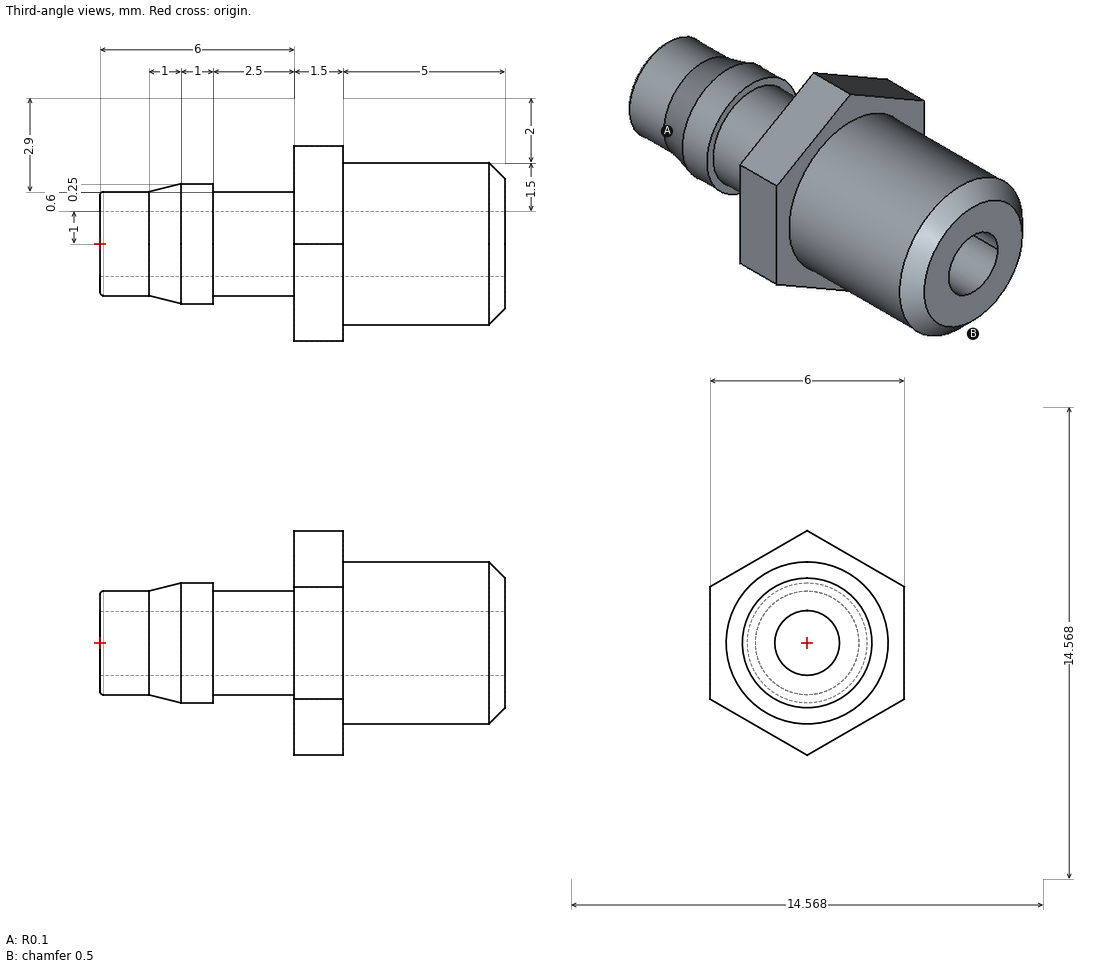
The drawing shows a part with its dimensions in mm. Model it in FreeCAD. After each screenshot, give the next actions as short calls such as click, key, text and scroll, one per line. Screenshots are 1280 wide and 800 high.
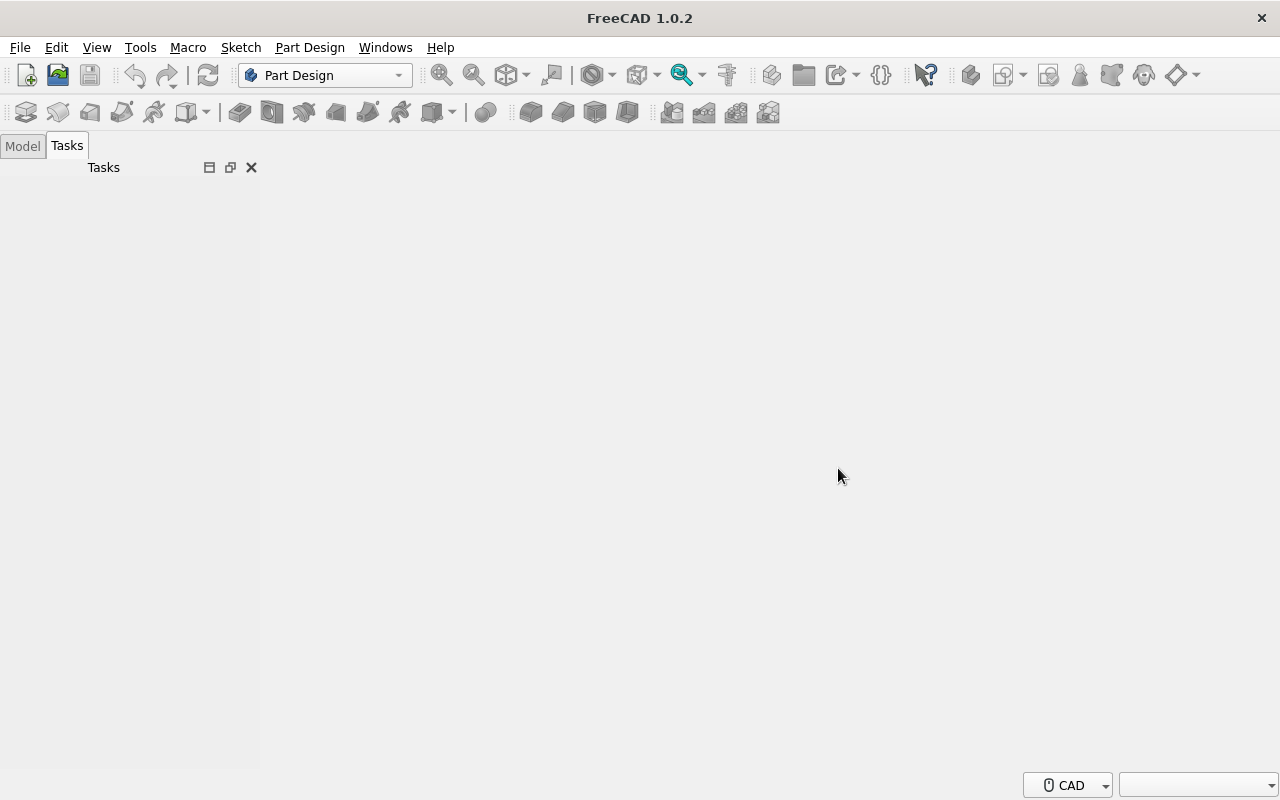
key(ctrl+n)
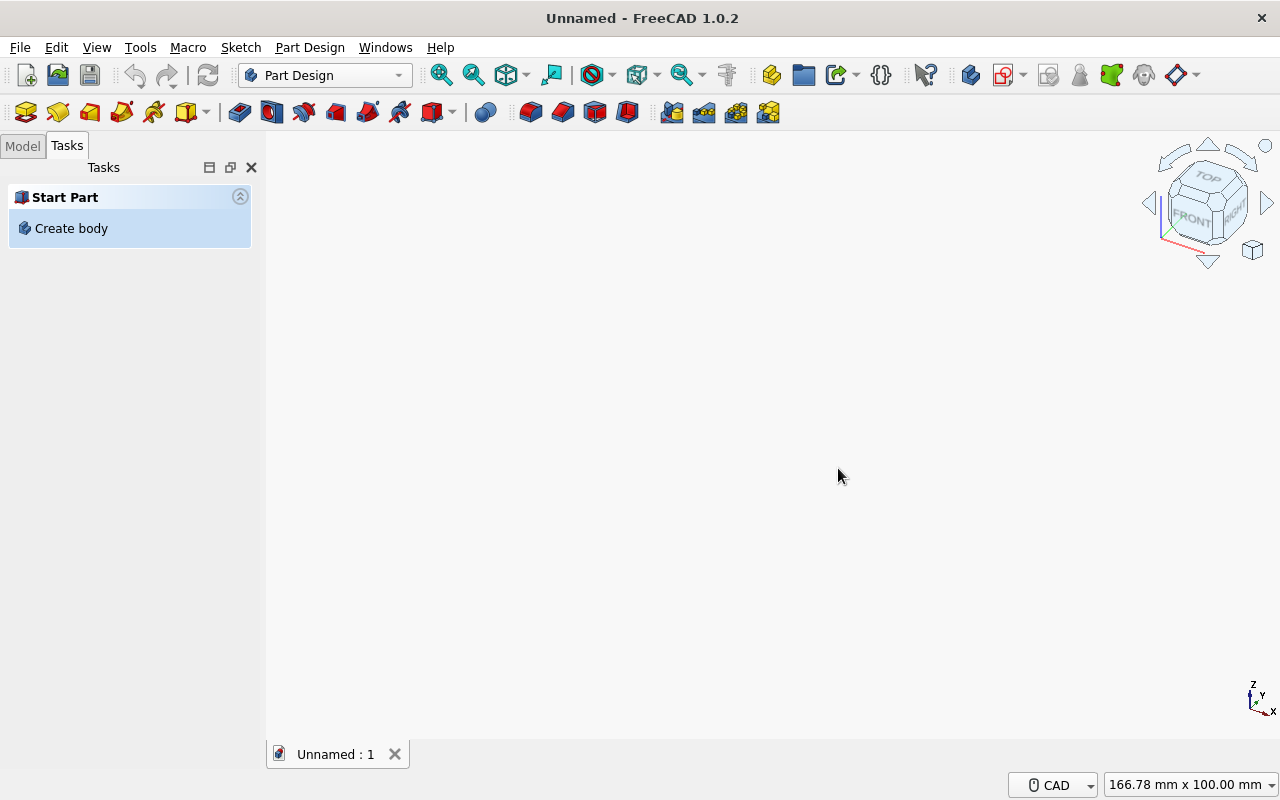
click(1004, 76)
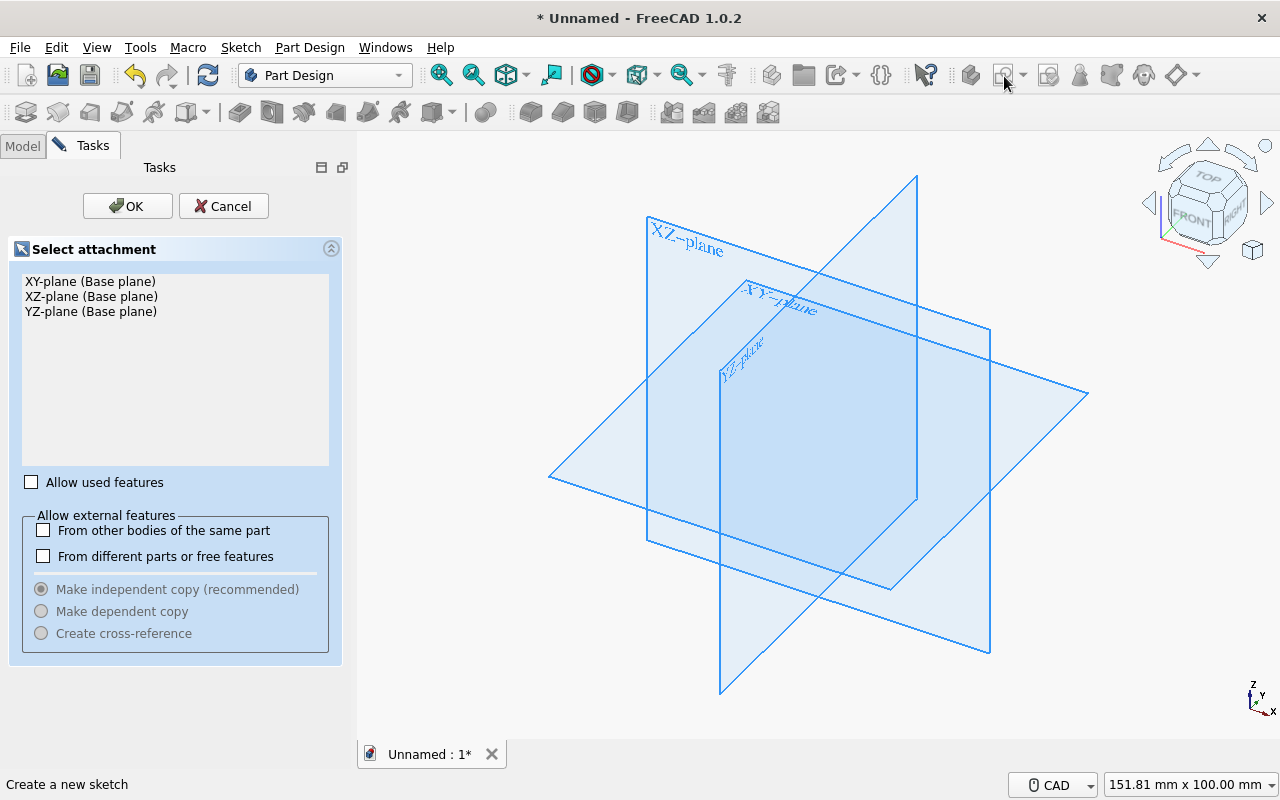
click(82, 282)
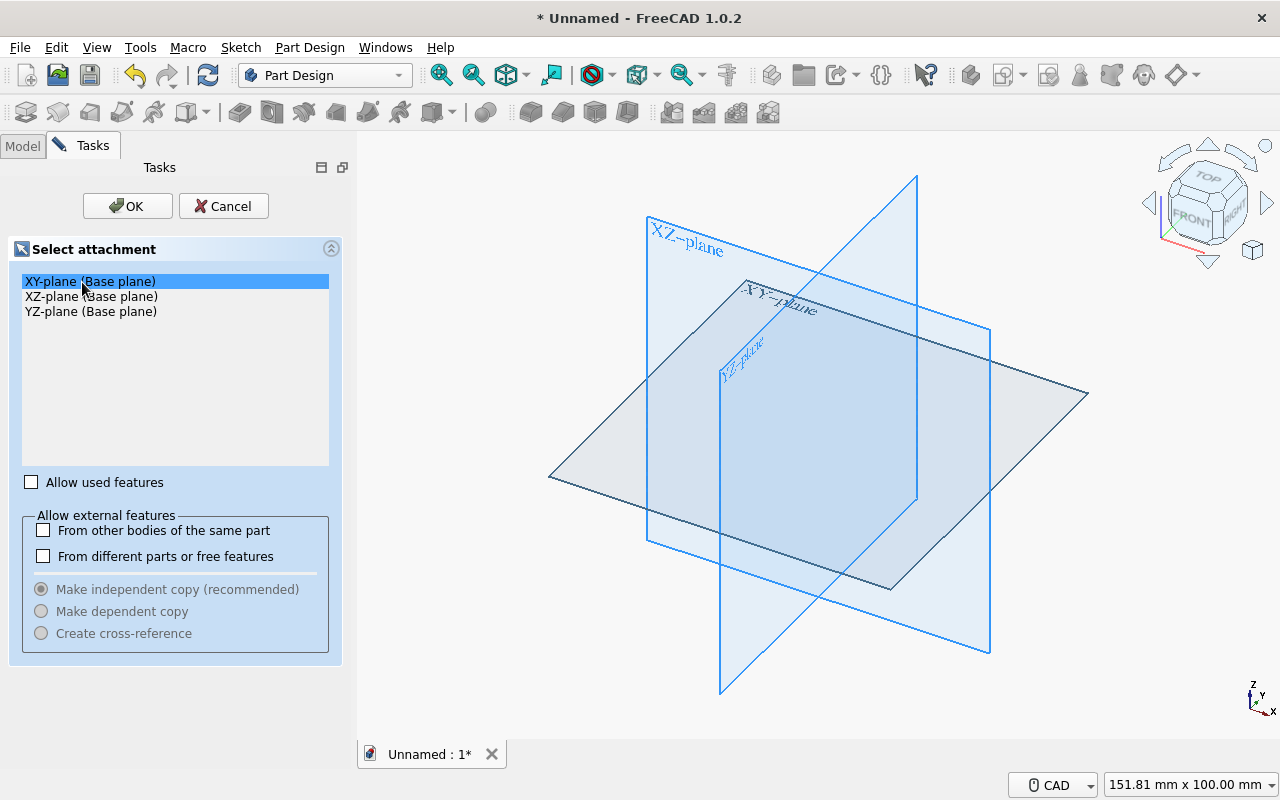
click(128, 206)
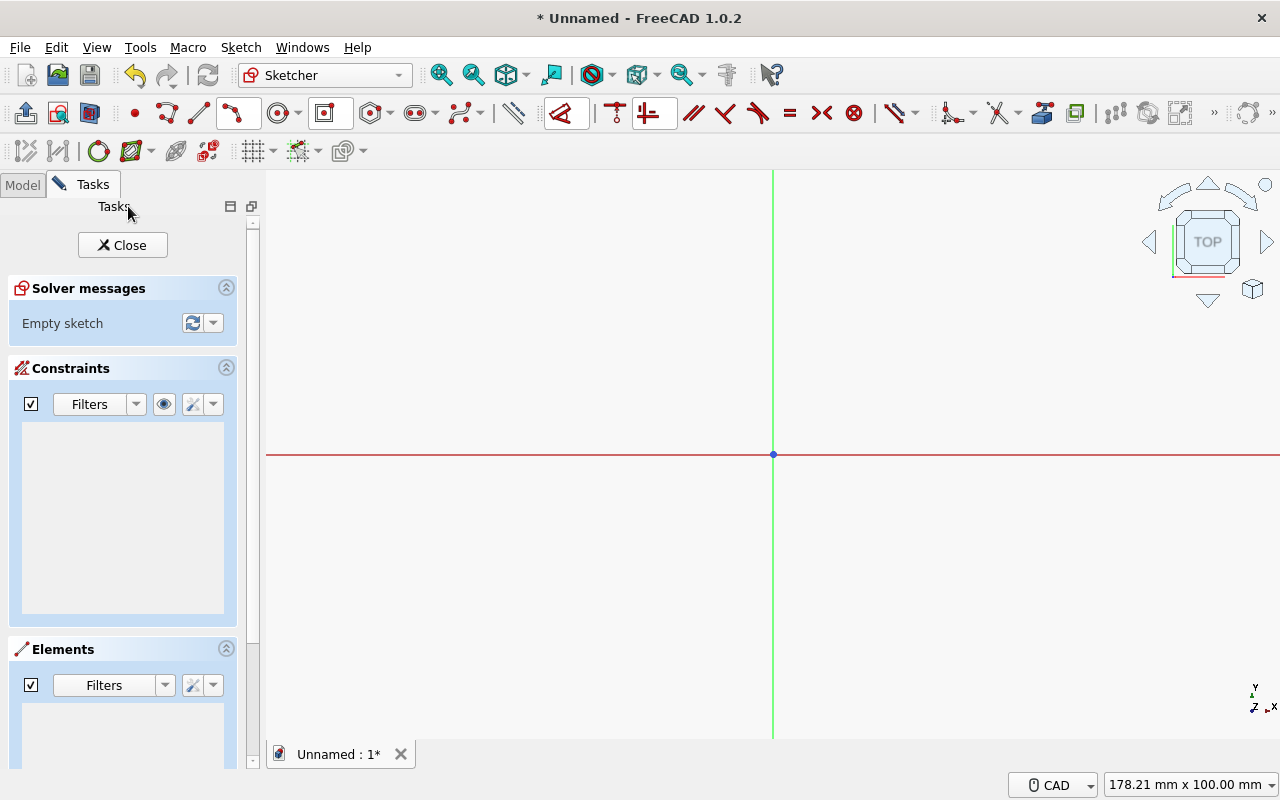
scroll(825, 440, up, 10)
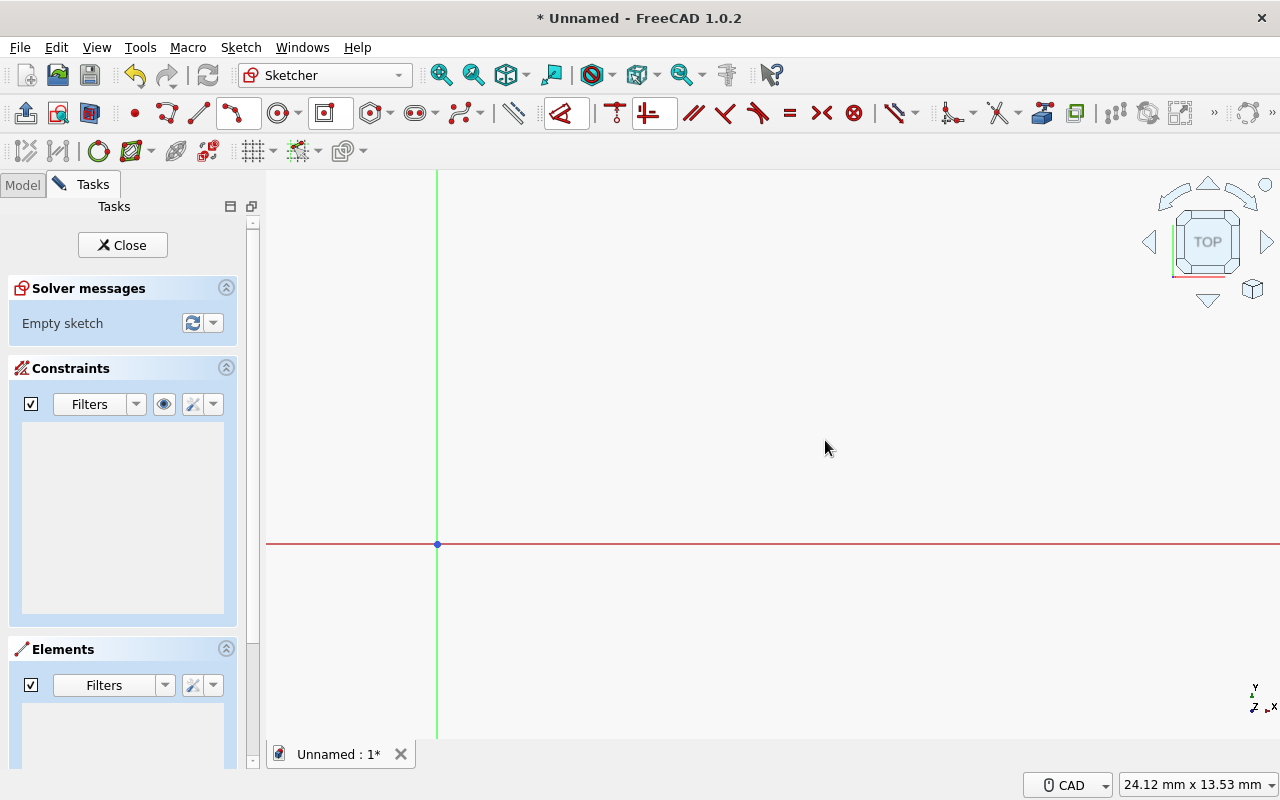
key(g)
key(m)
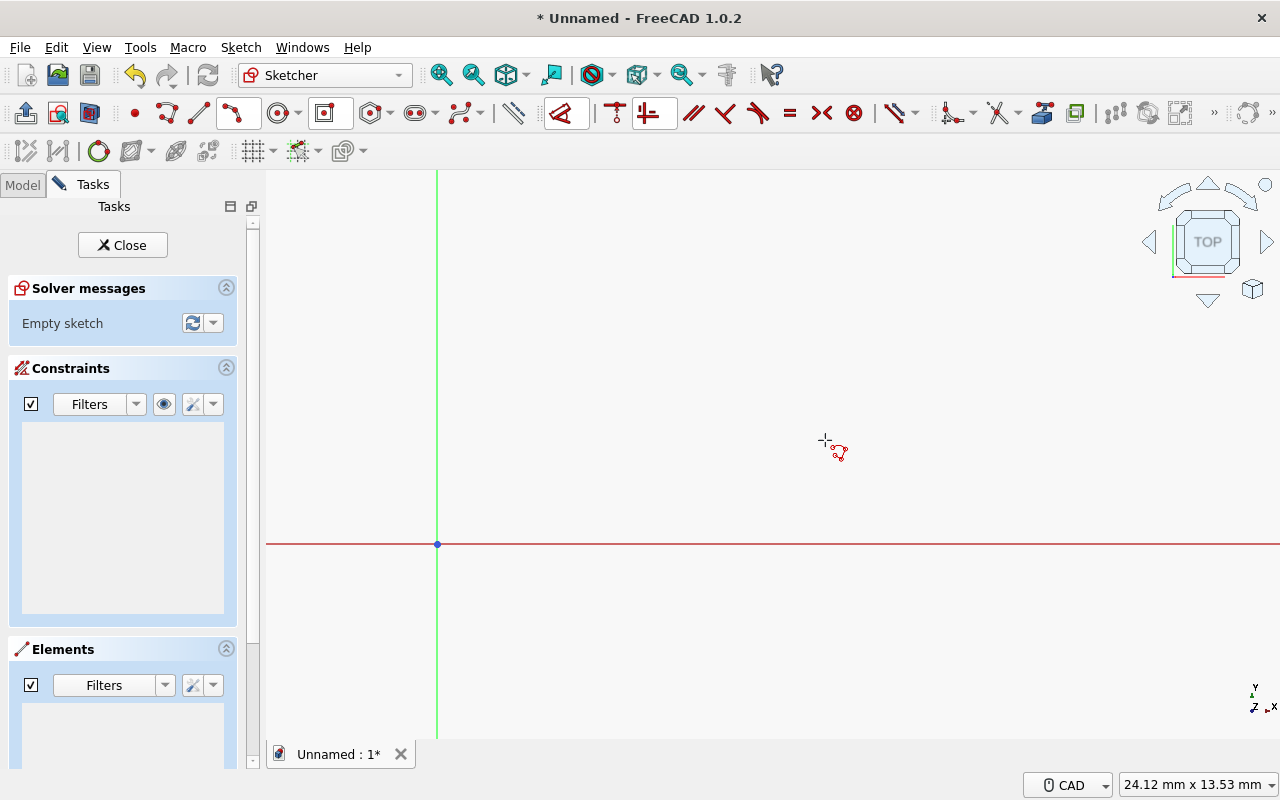
click(437, 502)
click(963, 502)
click(963, 439)
click(753, 439)
click(753, 355)
click(690, 355)
click(690, 477)
click(584, 477)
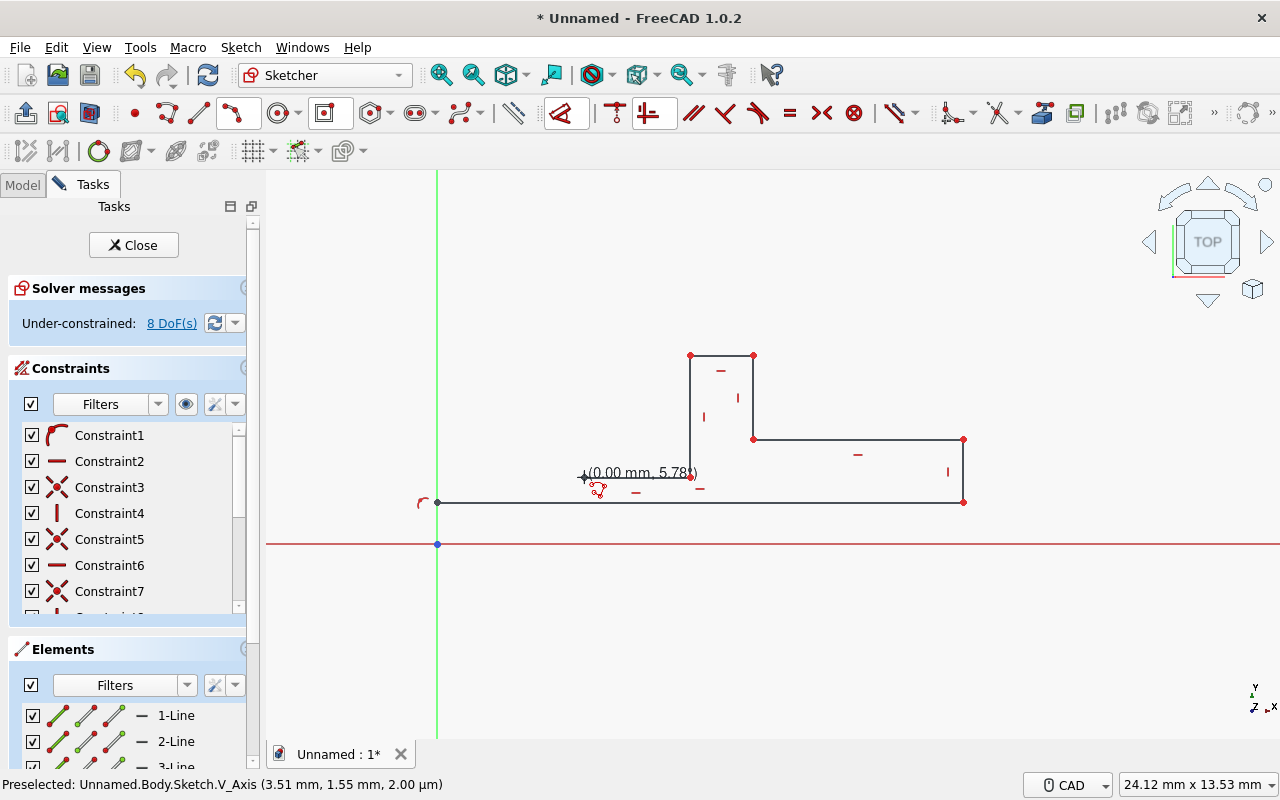
scroll(584, 466, up, 3)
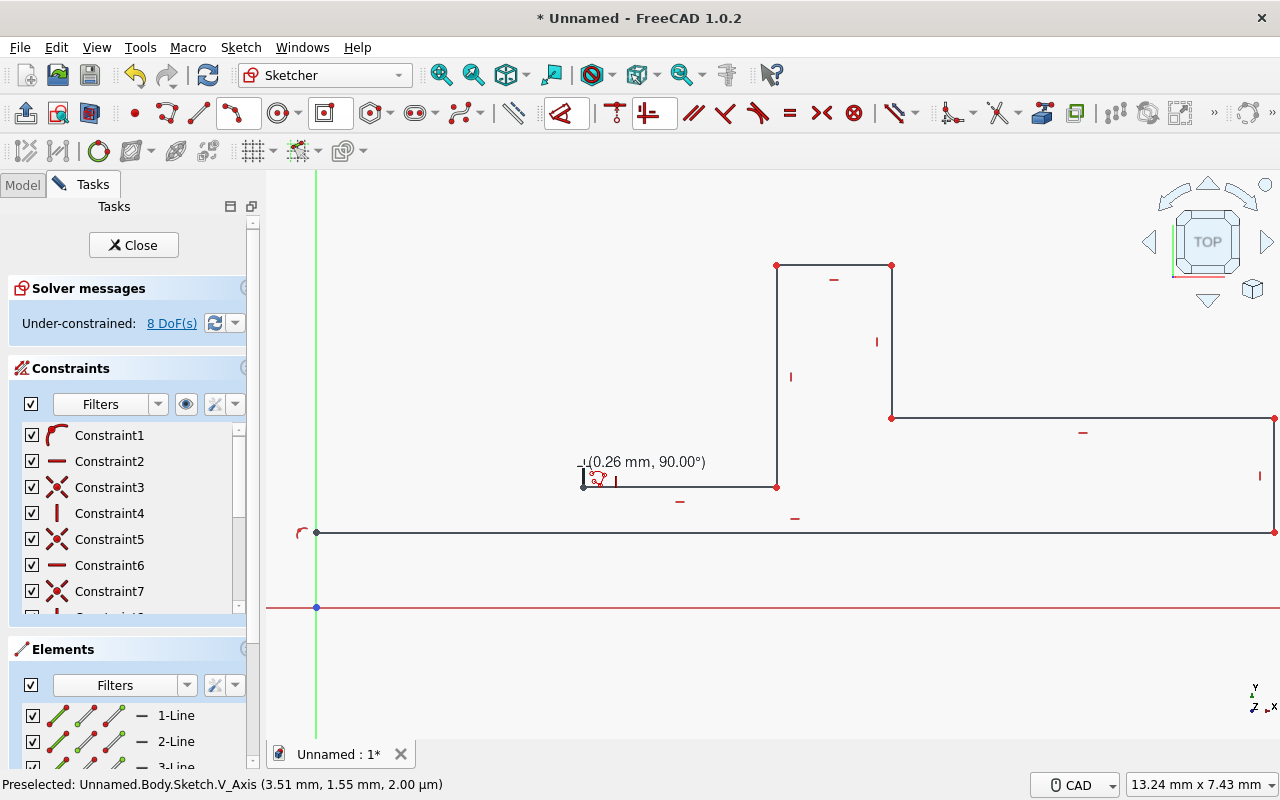
click(584, 466)
click(508, 466)
click(431, 485)
click(325, 485)
click(316, 533)
key(Escape)
key(Escape)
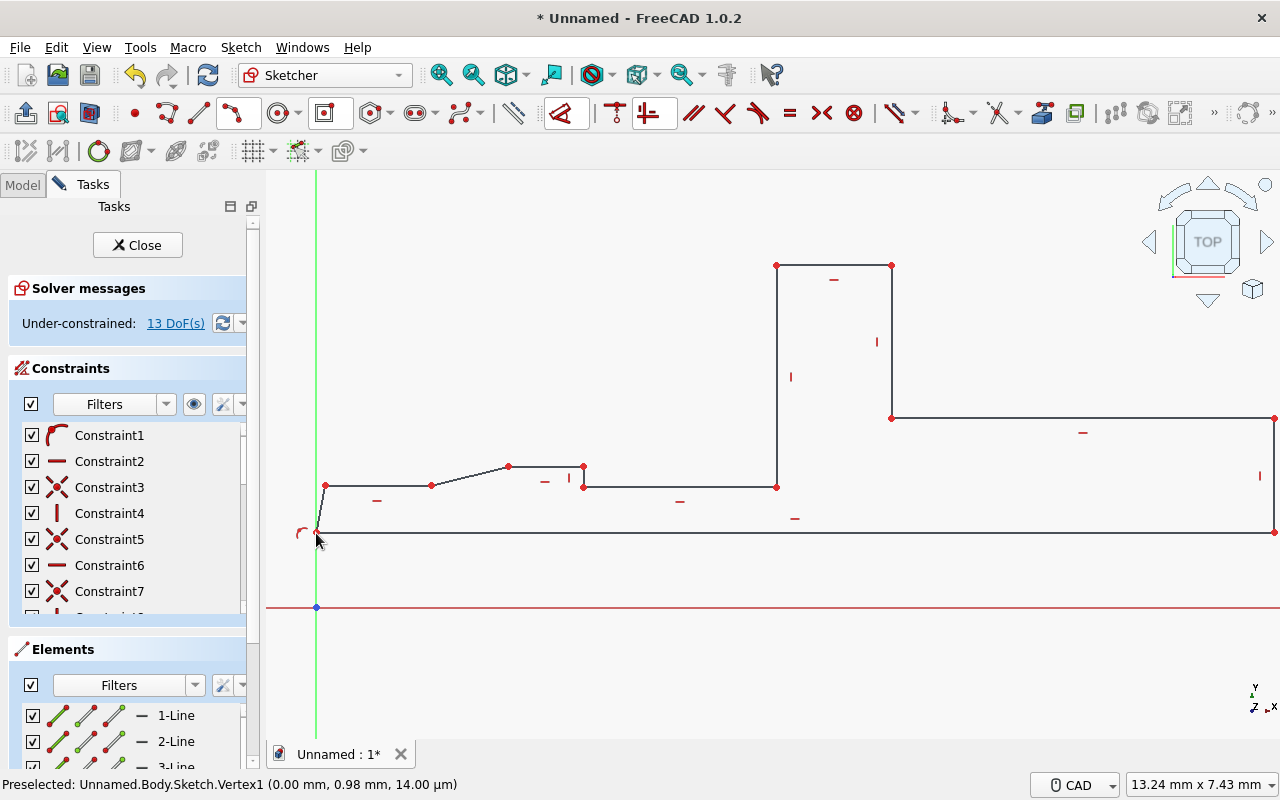
click(319, 519)